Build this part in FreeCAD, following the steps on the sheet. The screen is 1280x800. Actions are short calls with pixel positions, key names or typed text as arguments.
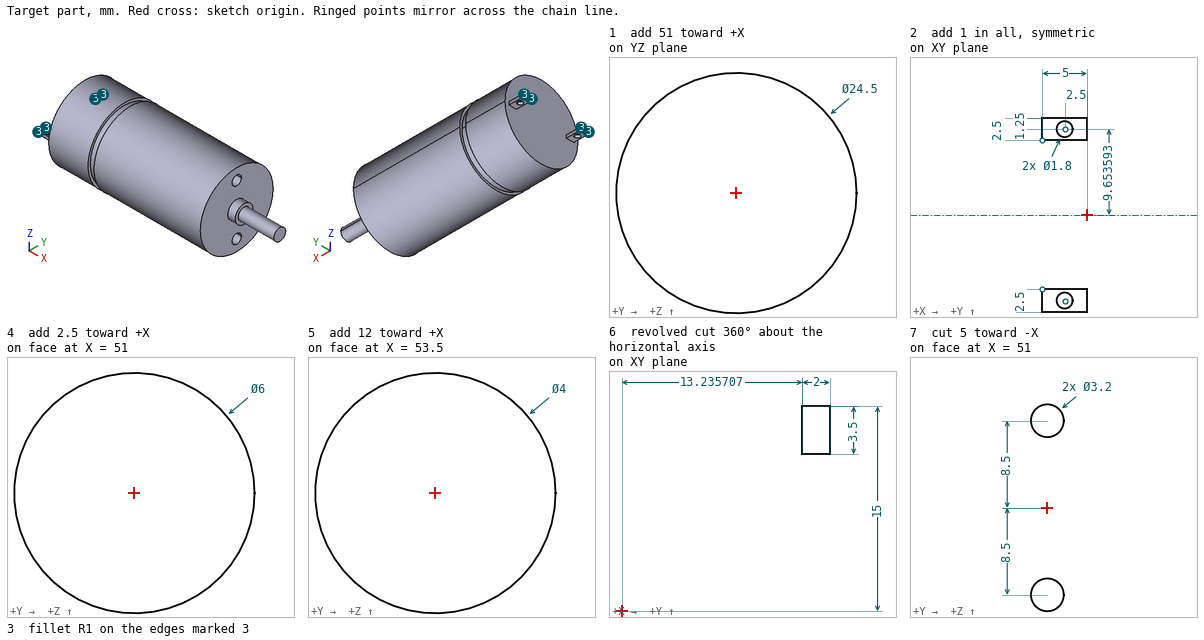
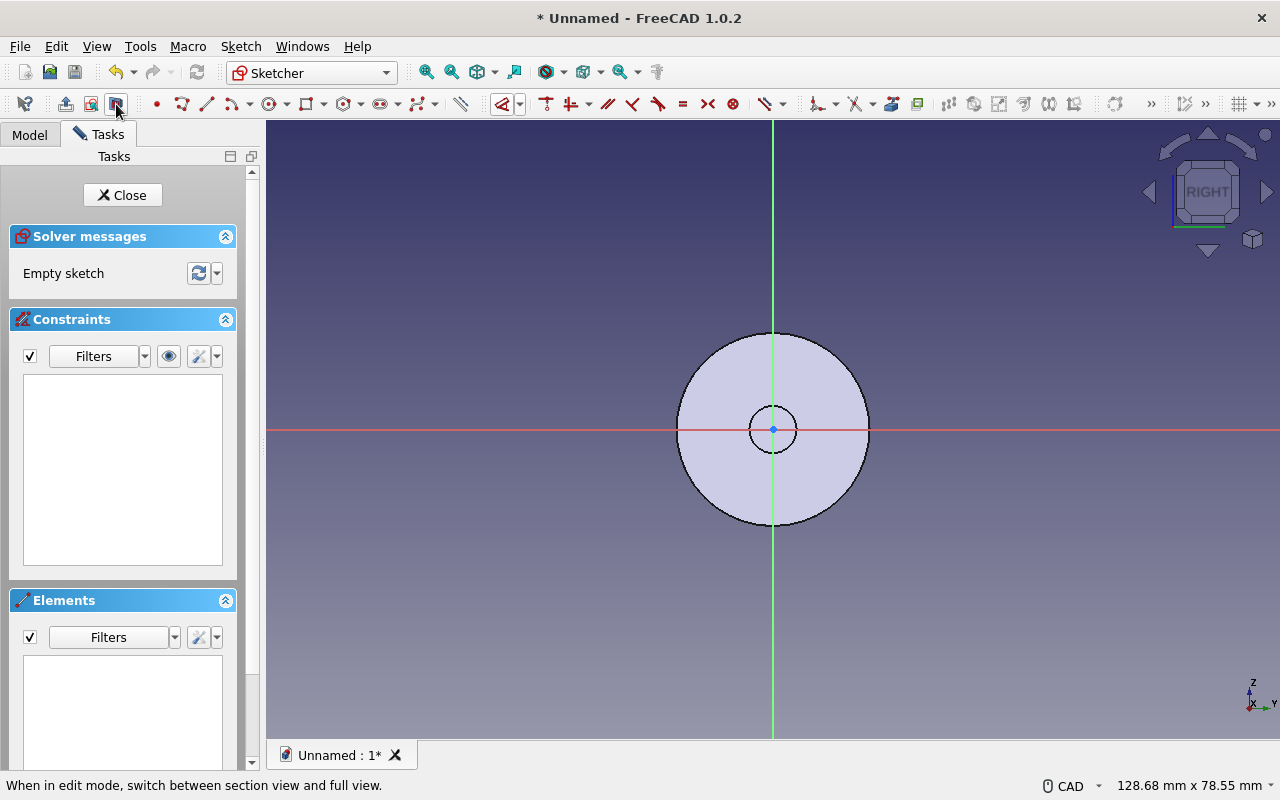
scroll(813, 429, up, 5)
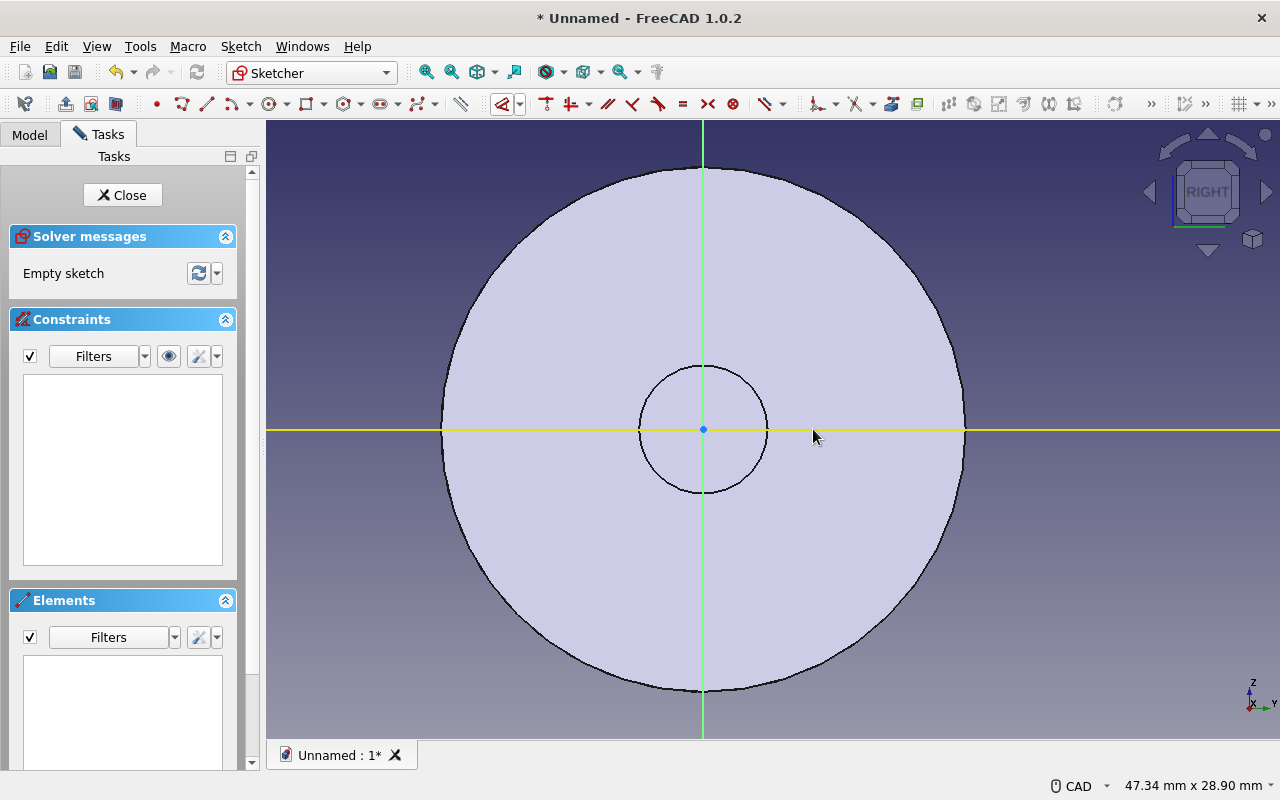
click(268, 104)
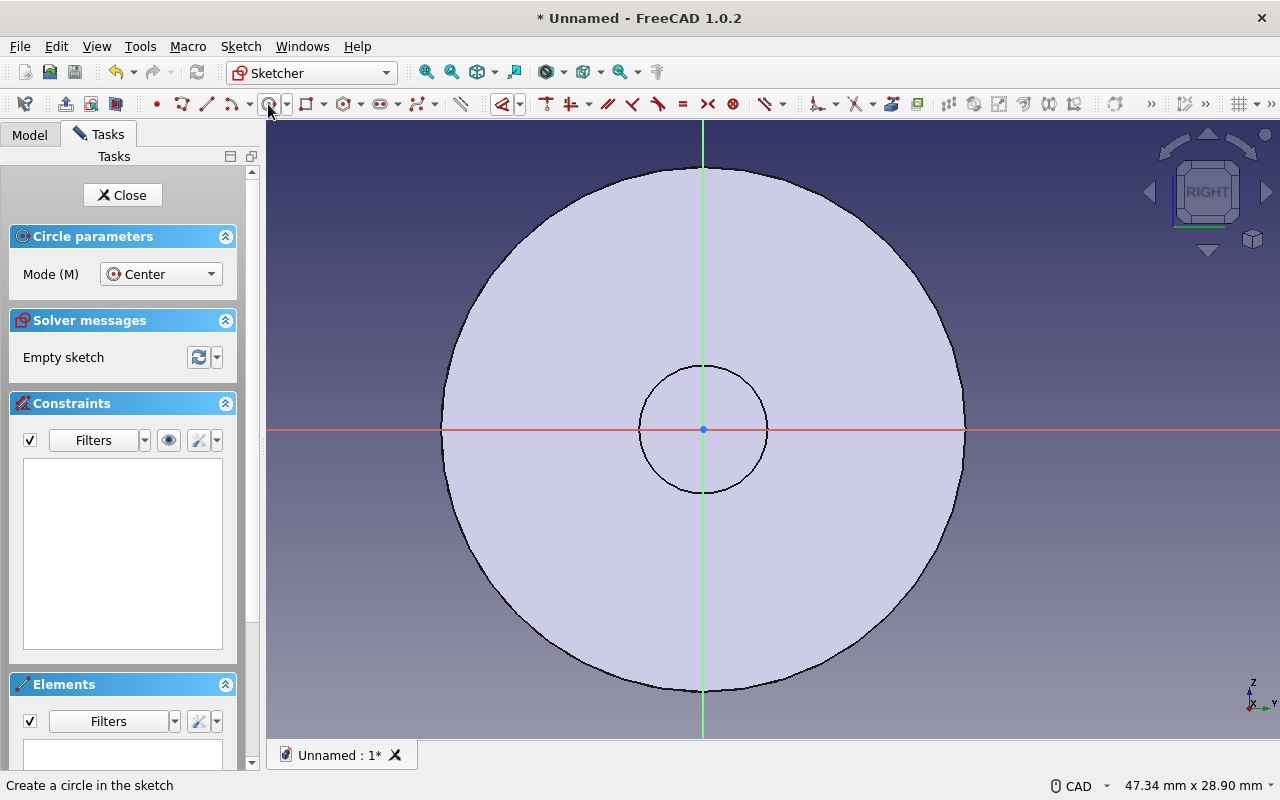
click(703, 247)
move(728, 223)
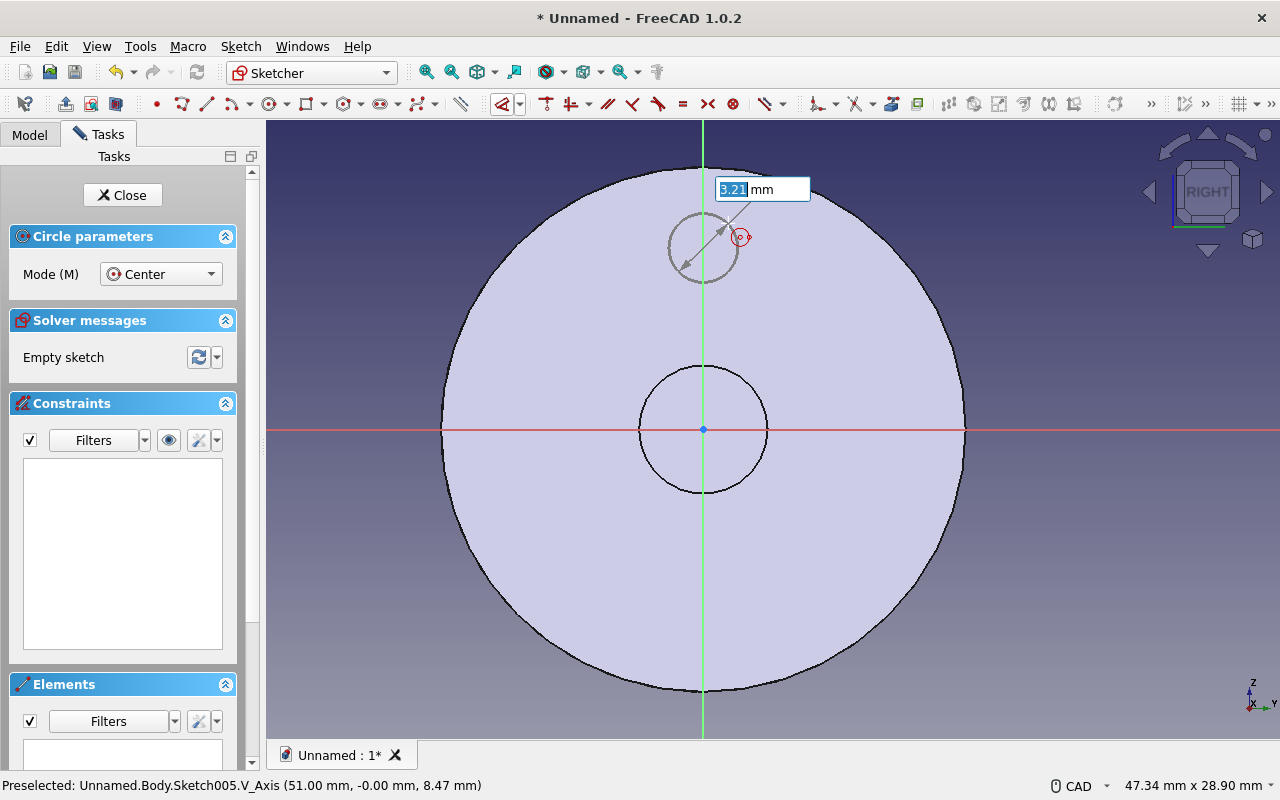
text(3.2)
key(Return)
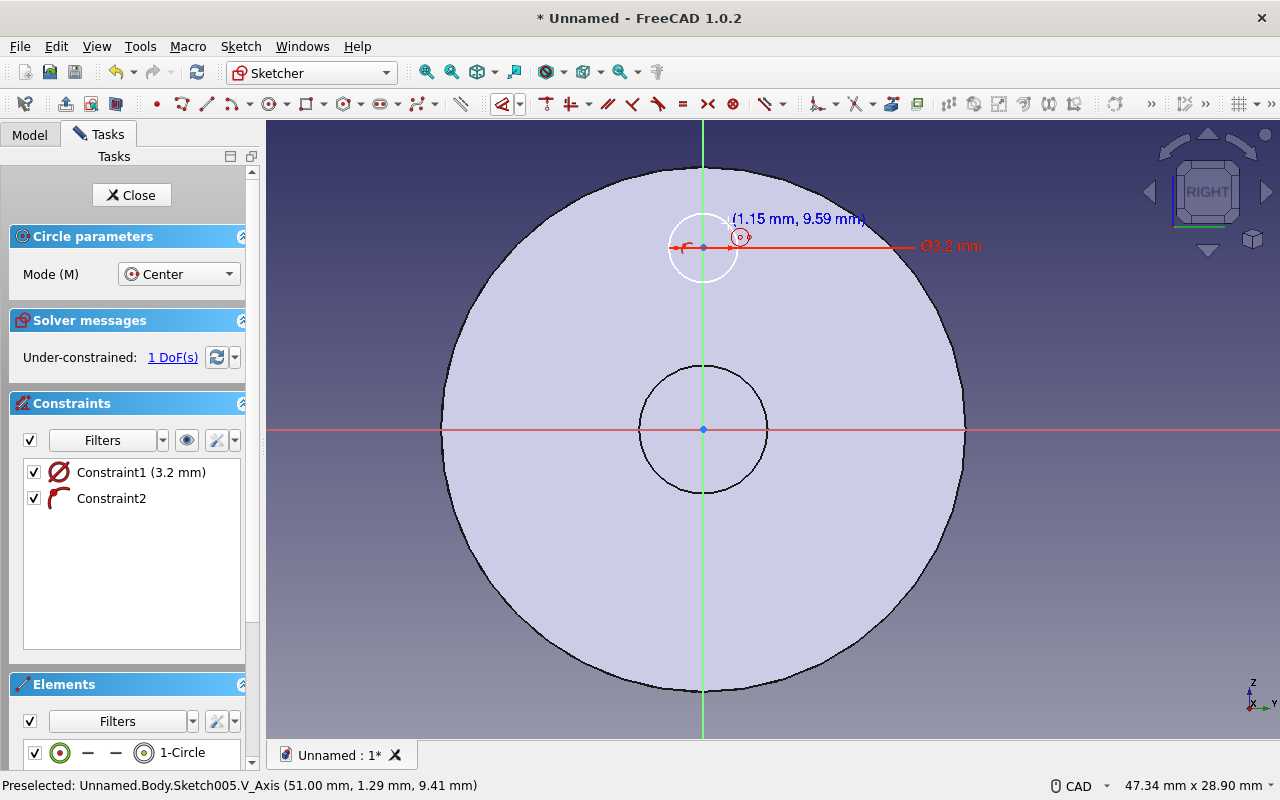
click(703, 612)
move(728, 587)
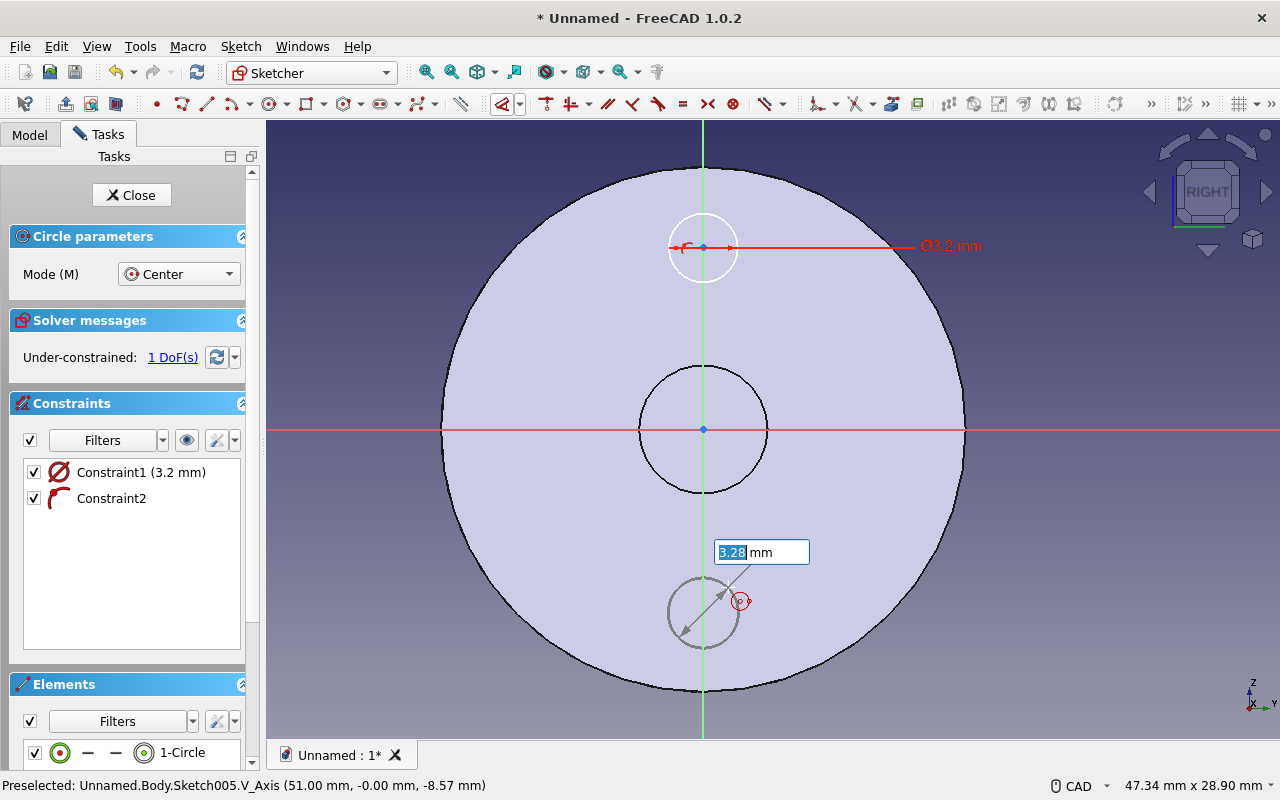
text(3.2)
key(Return)
key(Escape)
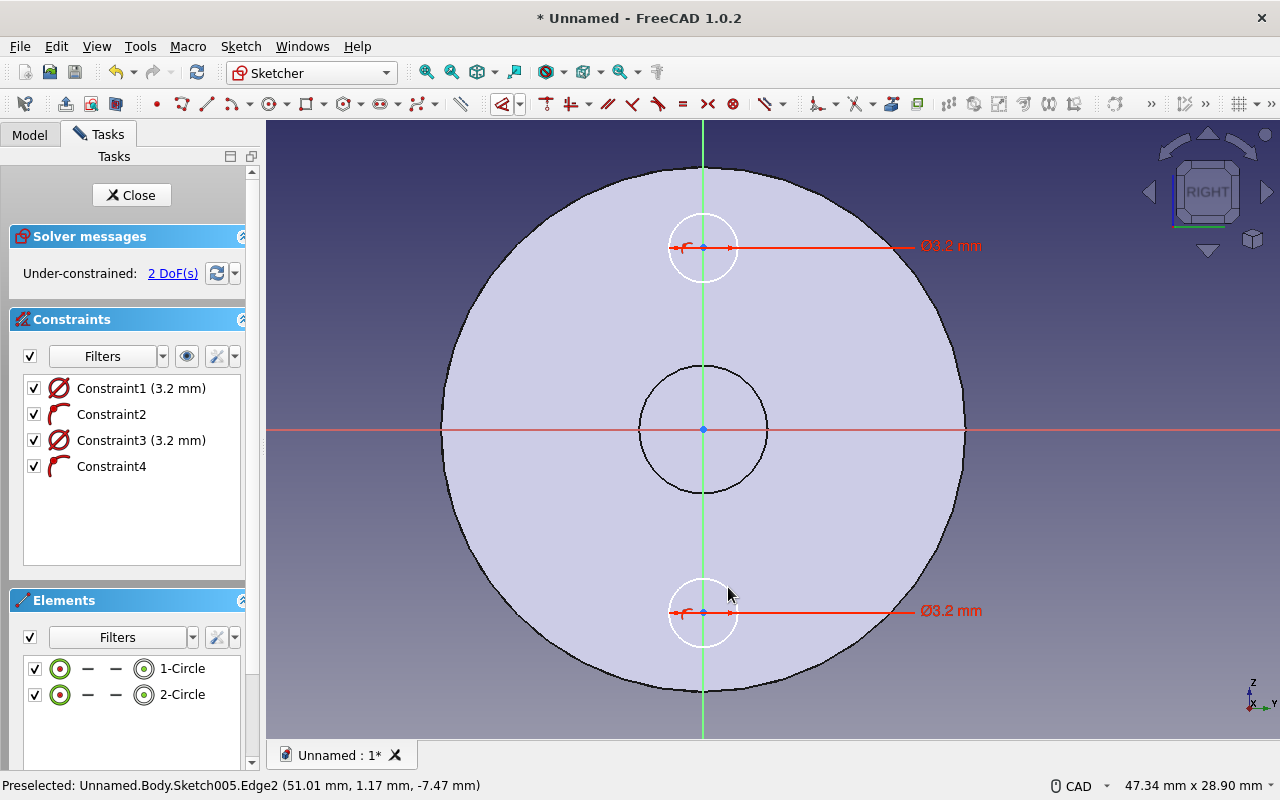
click(703, 248)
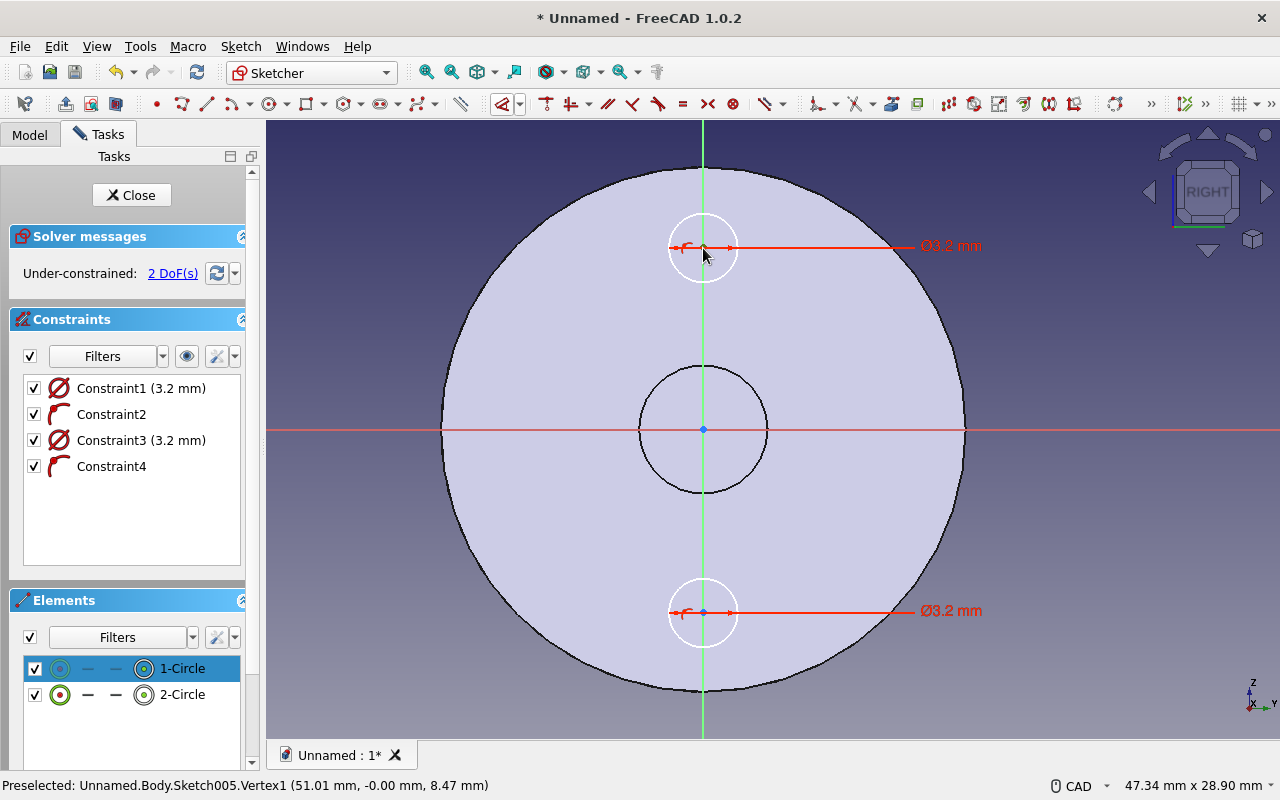
click(520, 104)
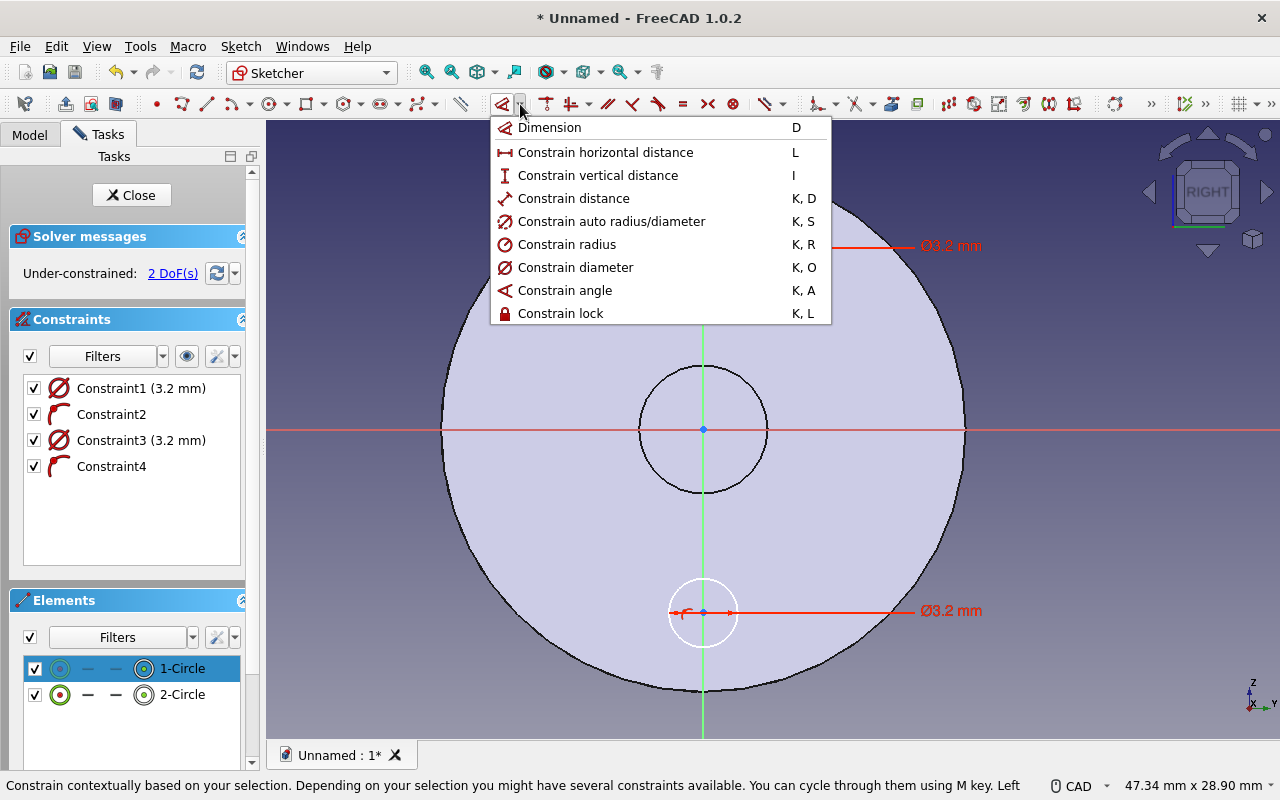
click(661, 176)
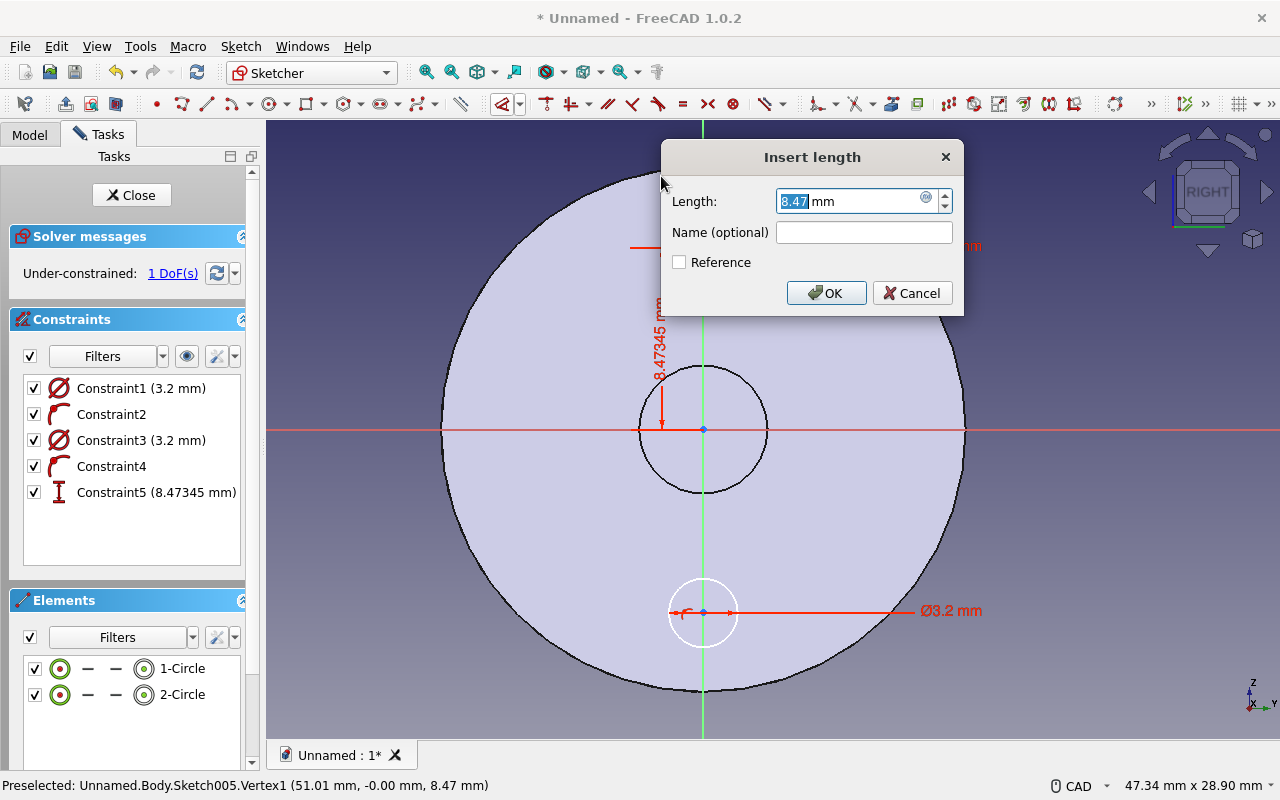
text(8.5)
key(Return)